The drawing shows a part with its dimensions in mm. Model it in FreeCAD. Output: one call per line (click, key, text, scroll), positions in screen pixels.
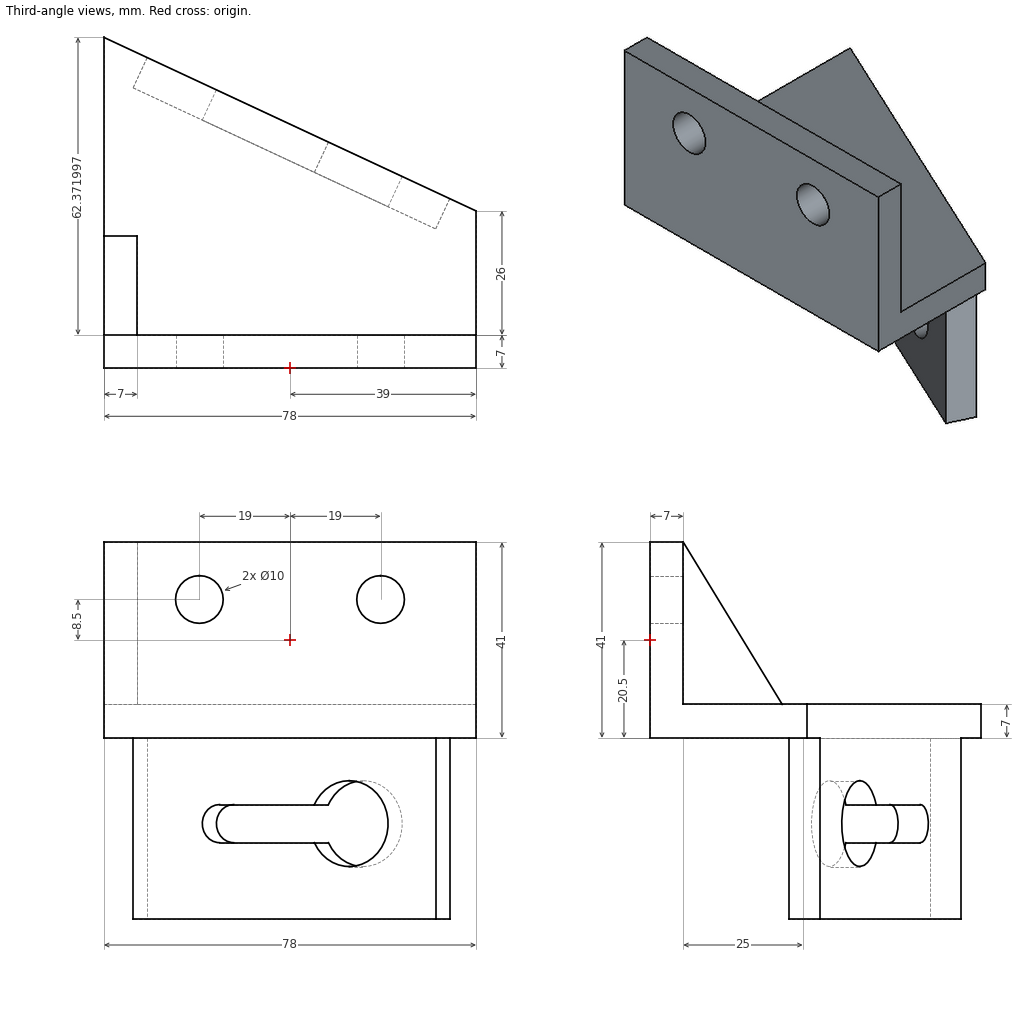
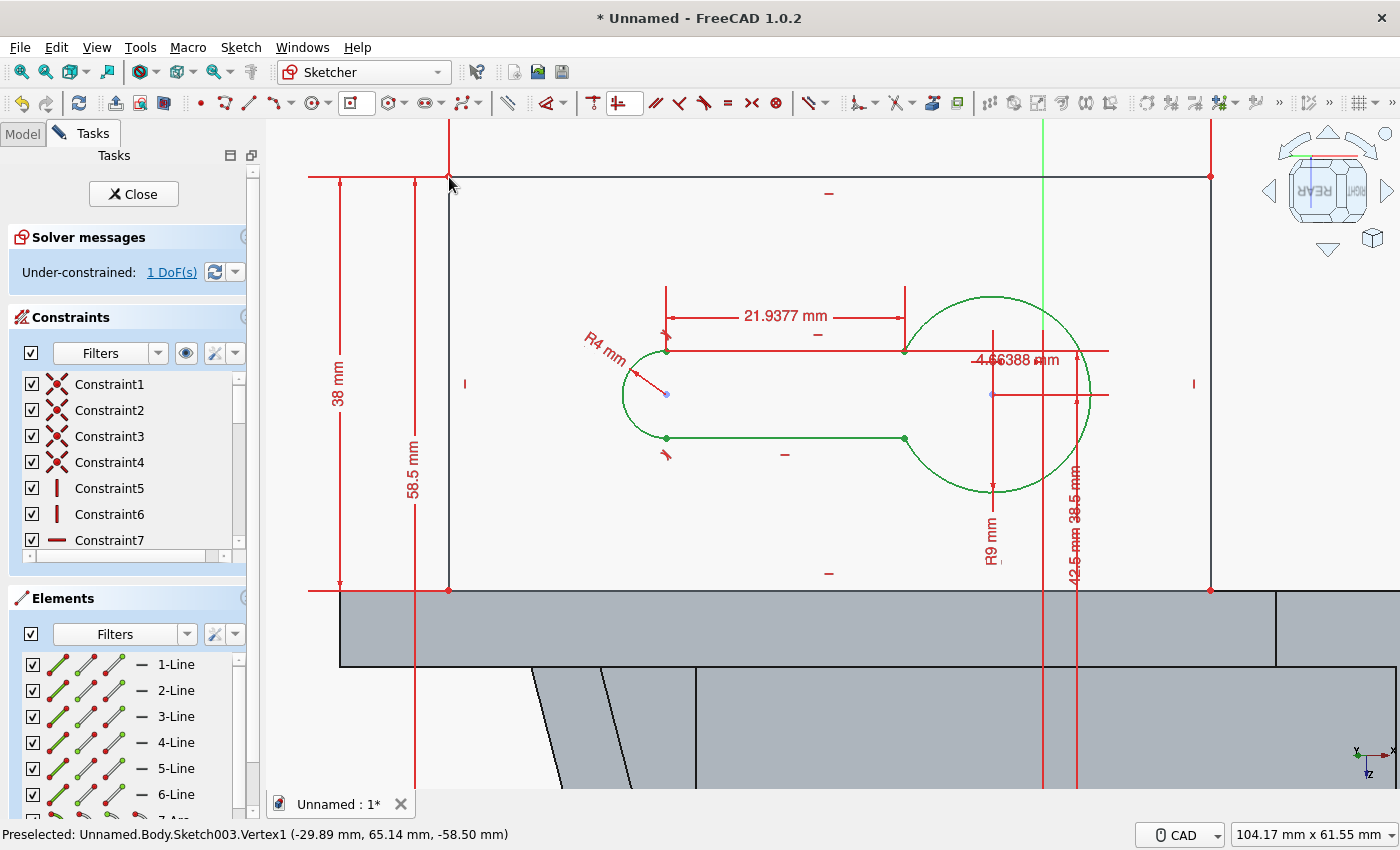
click(449, 177)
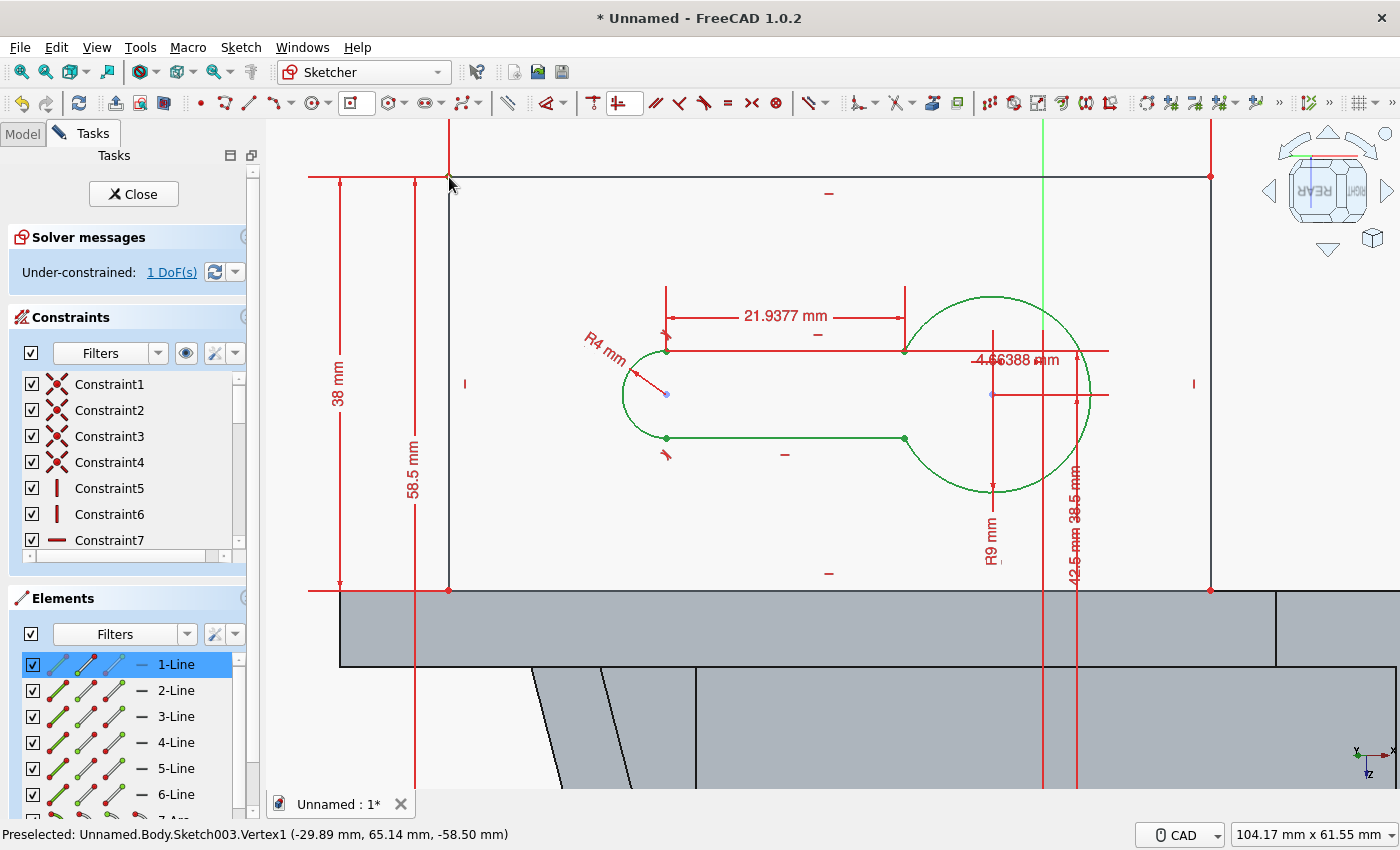
key(l)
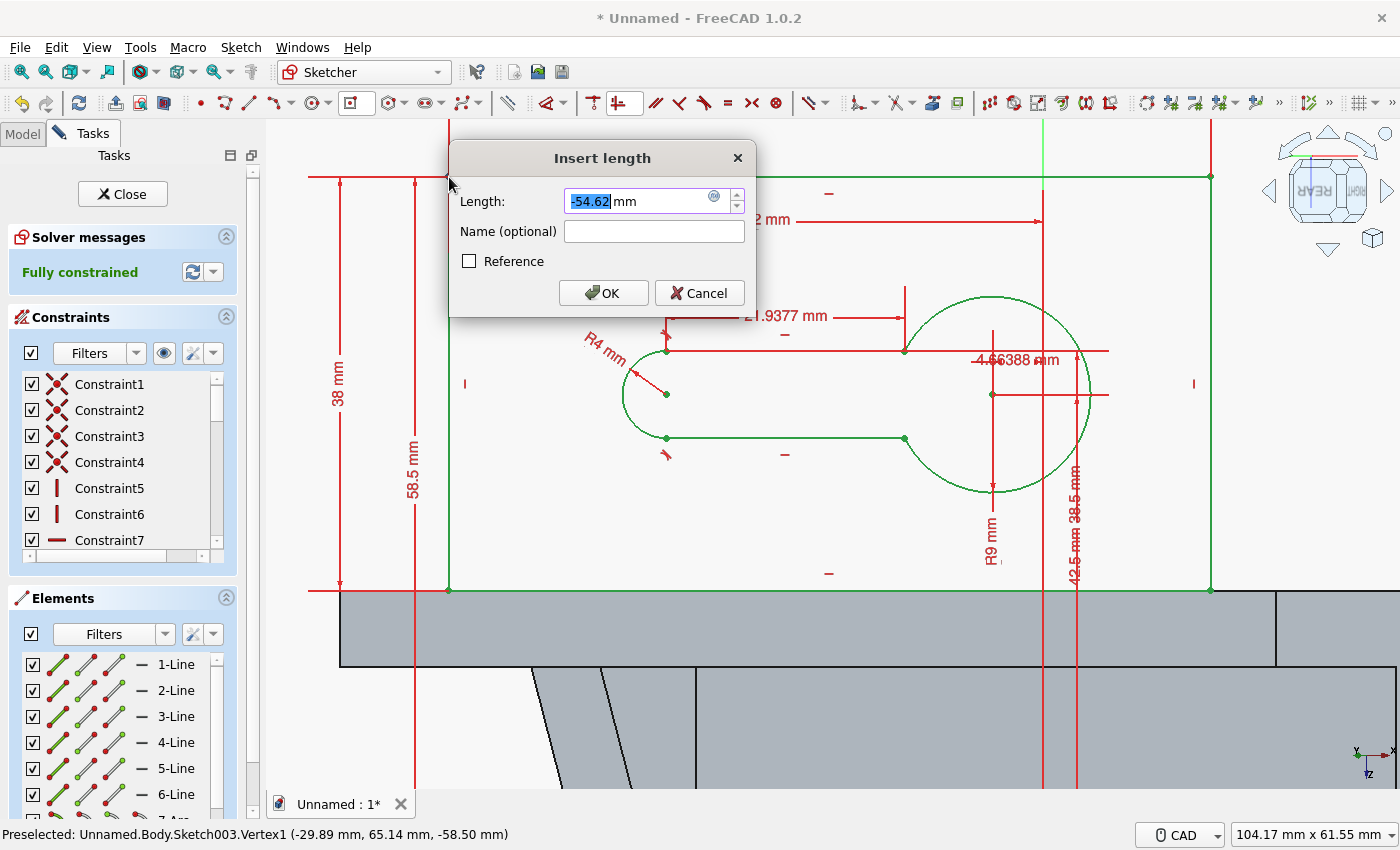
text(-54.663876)
key(Return)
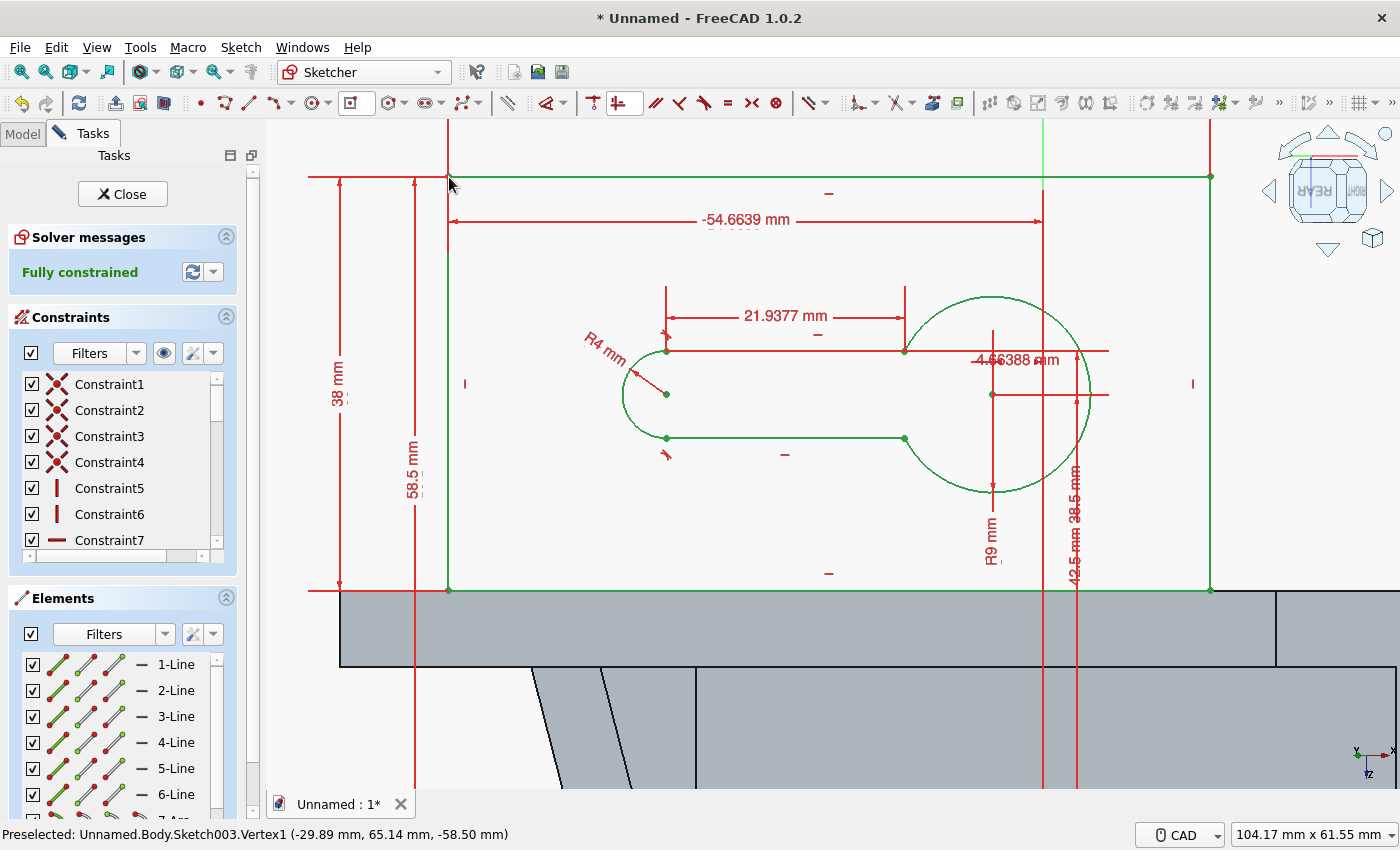
click(123, 194)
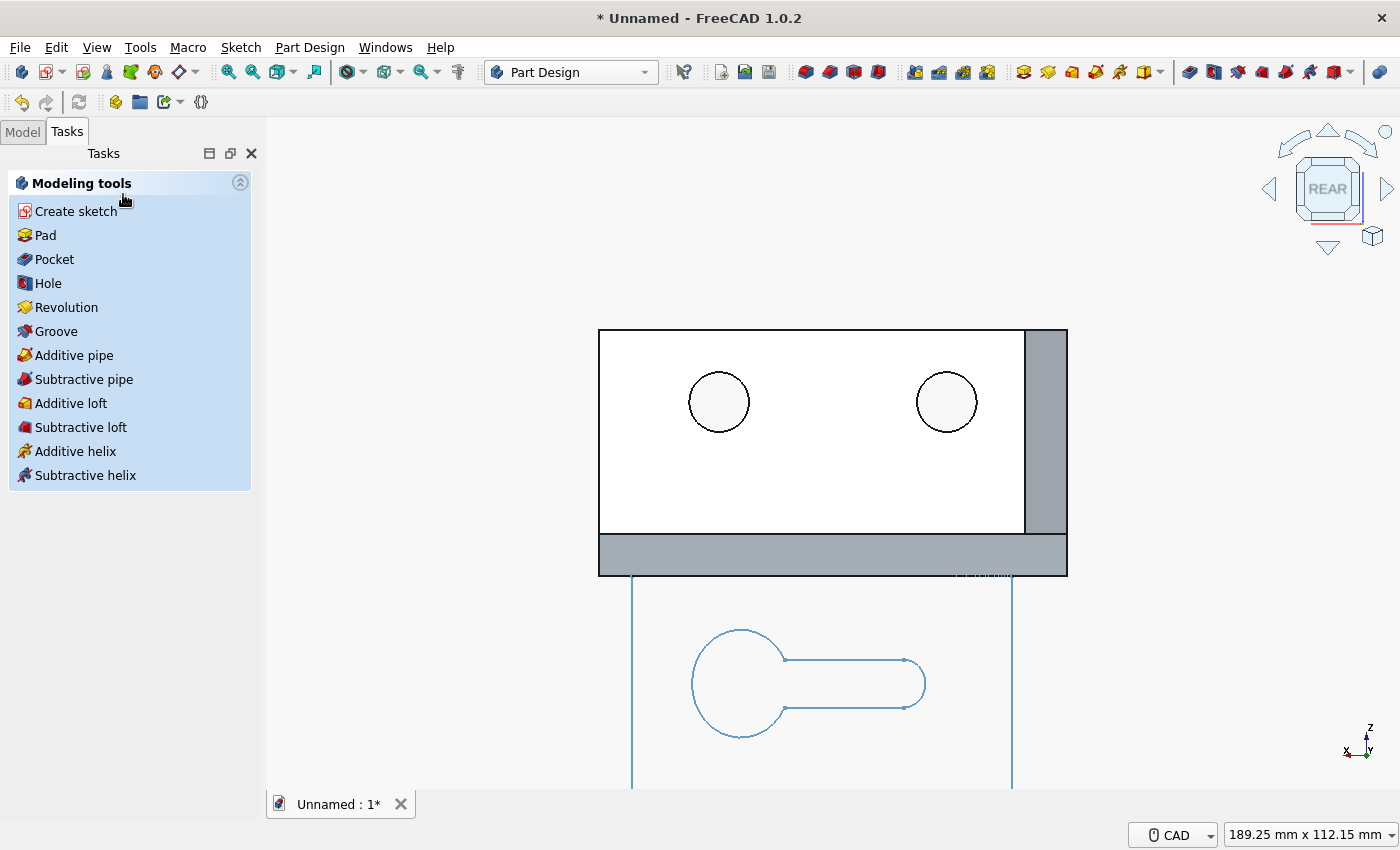
click(1024, 72)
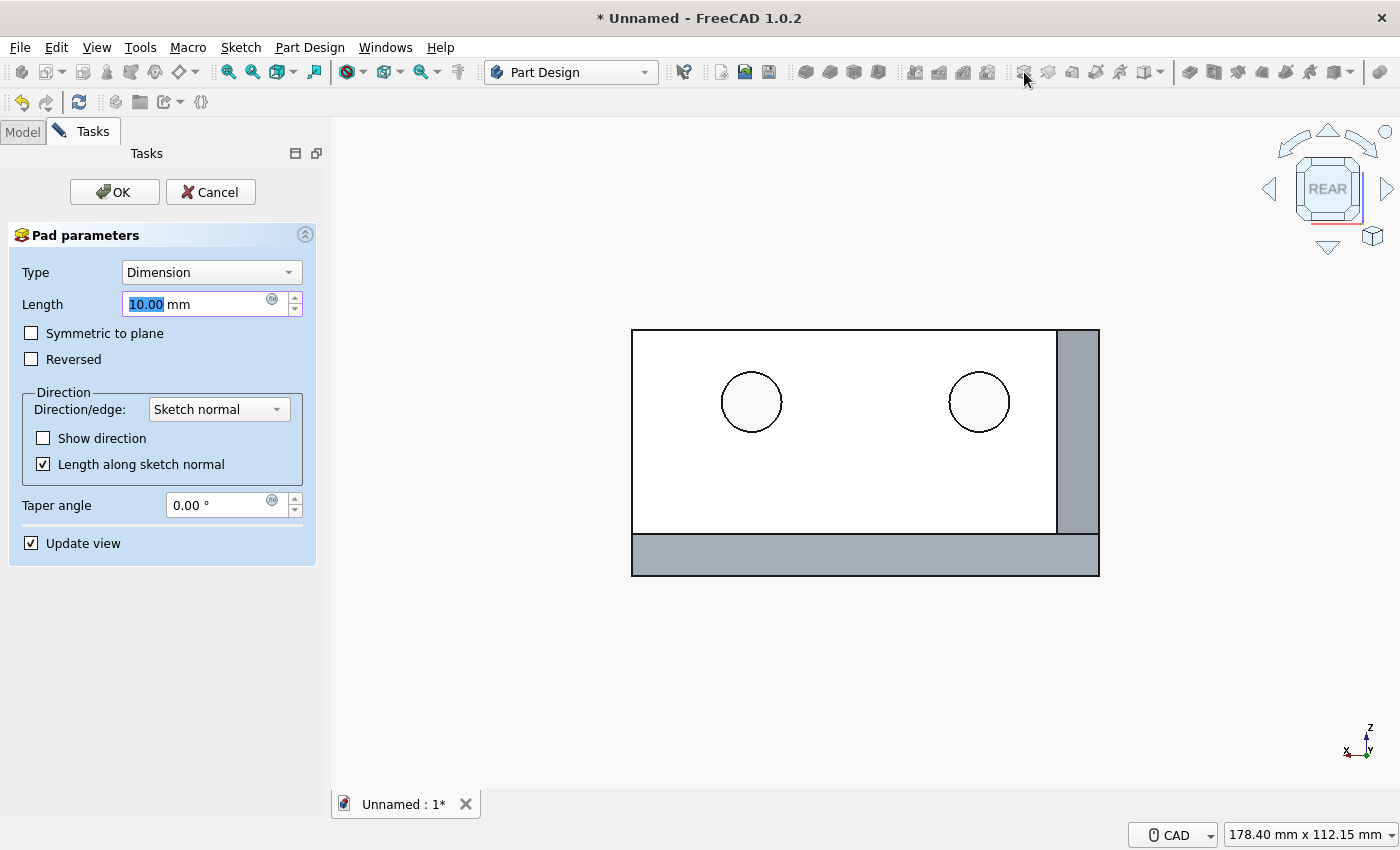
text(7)
key(Tab)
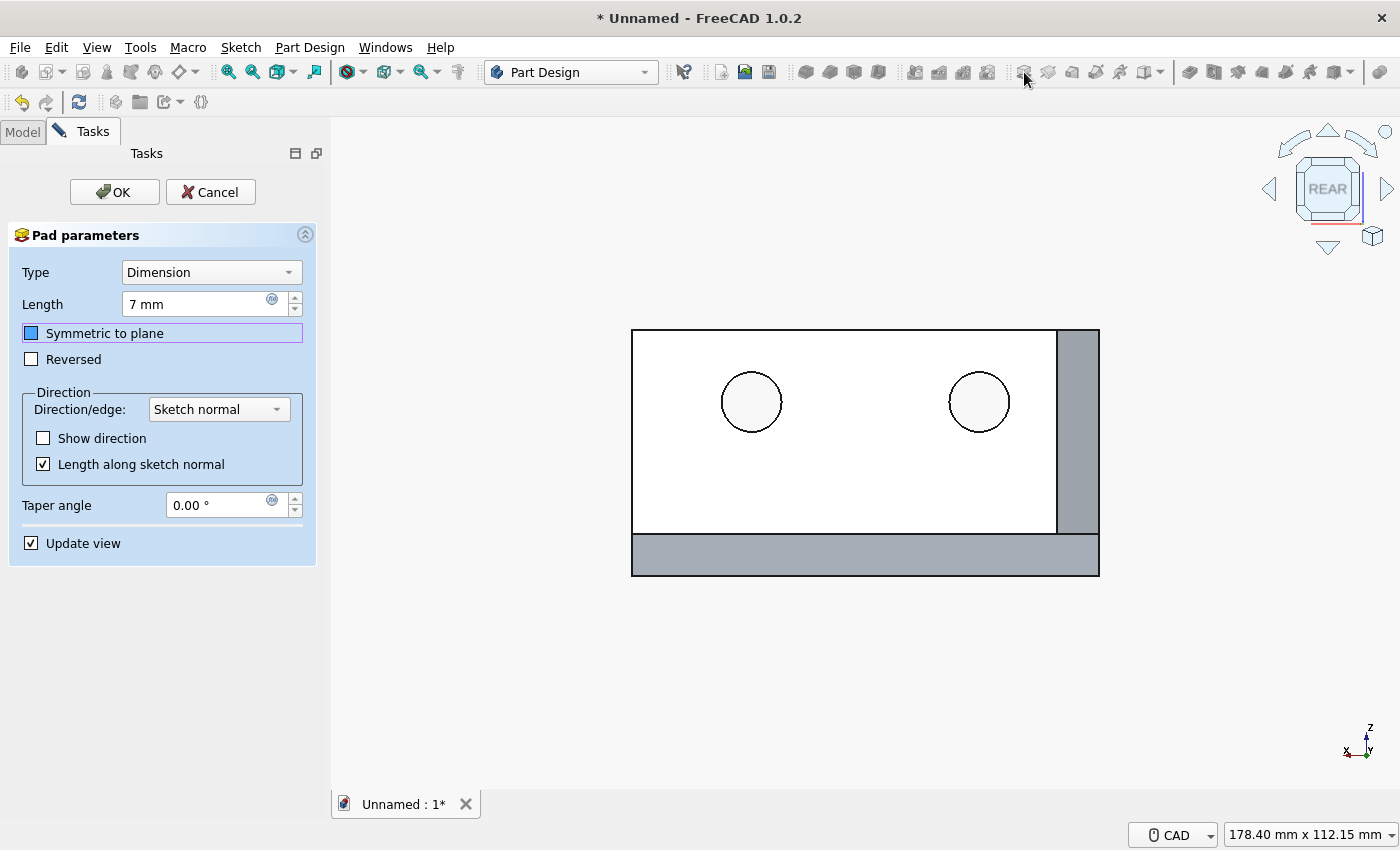
click(30, 359)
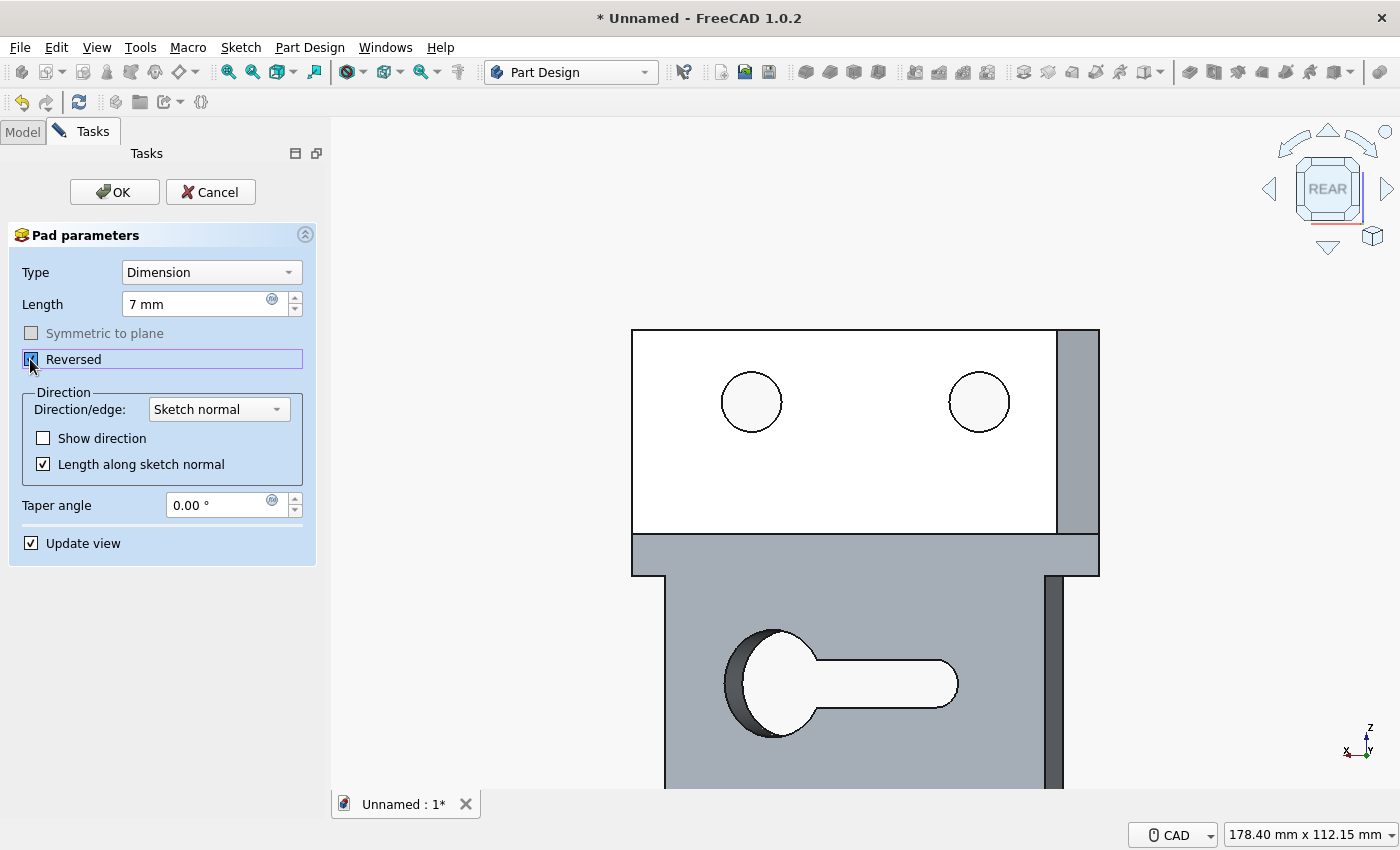
click(115, 192)